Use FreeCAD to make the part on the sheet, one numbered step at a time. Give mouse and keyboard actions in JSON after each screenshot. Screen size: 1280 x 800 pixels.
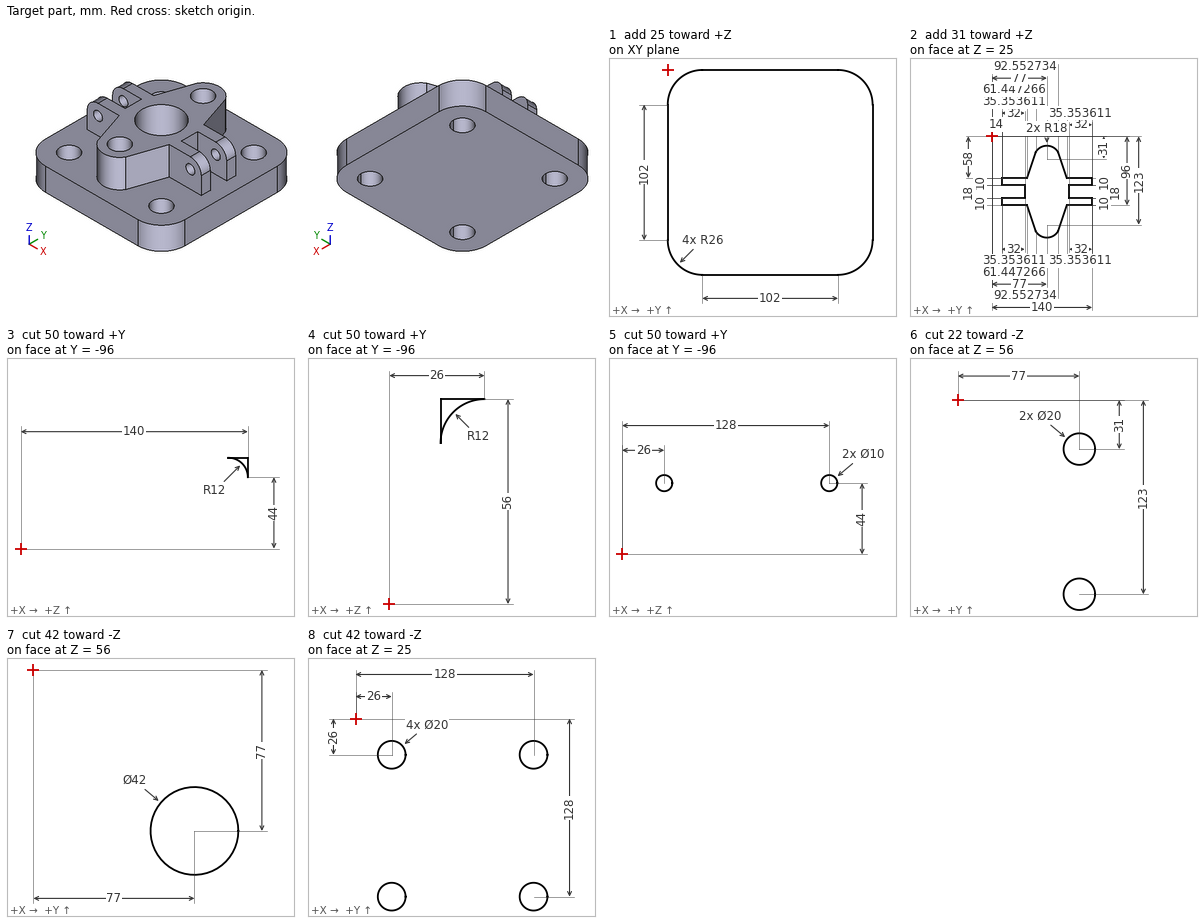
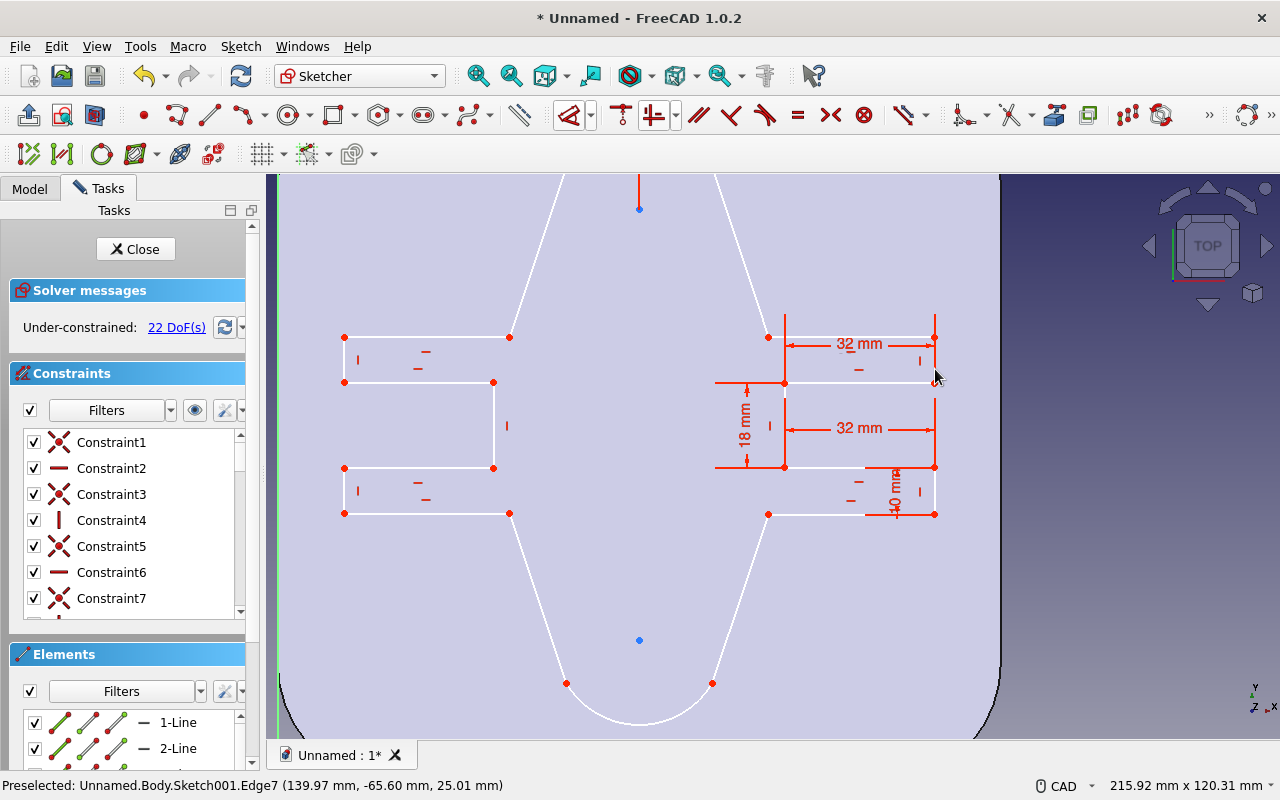
{"action": "left_click", "coordinate": [590, 116]}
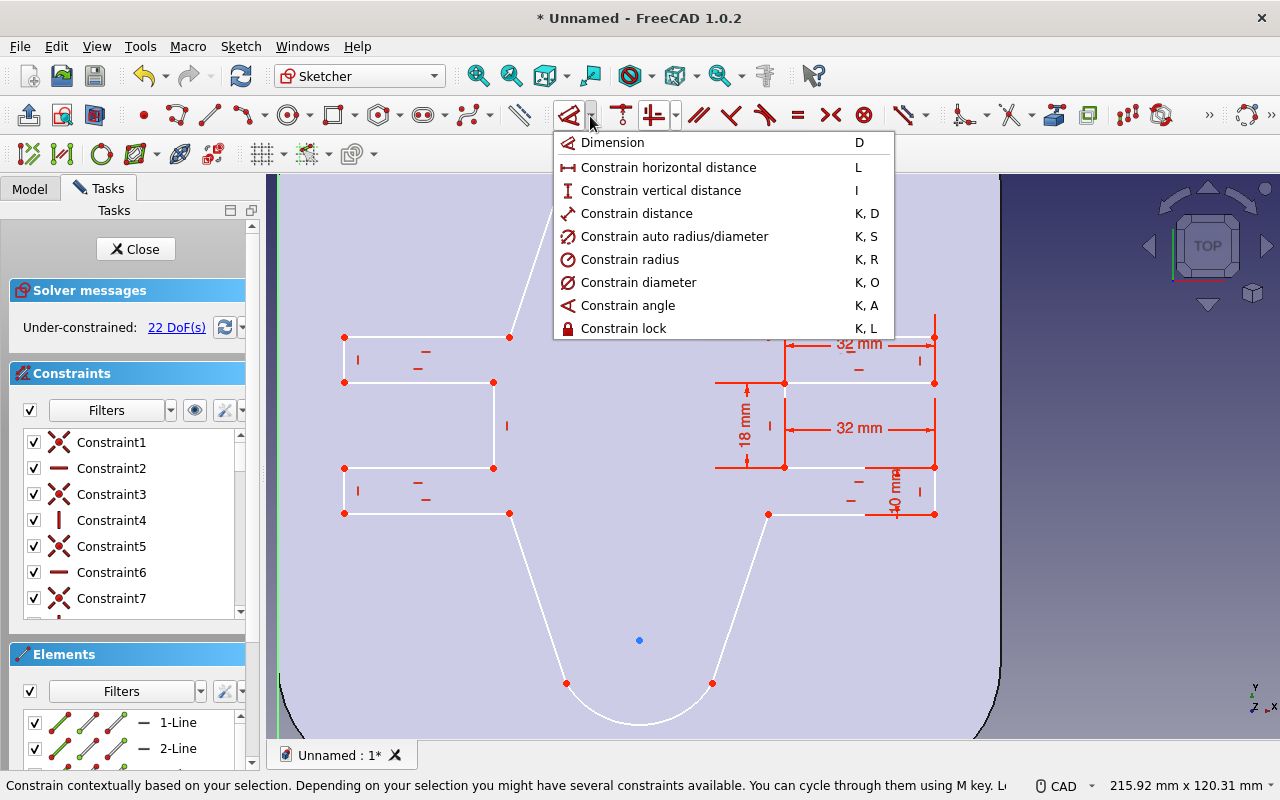
{"action": "left_click", "coordinate": [724, 190]}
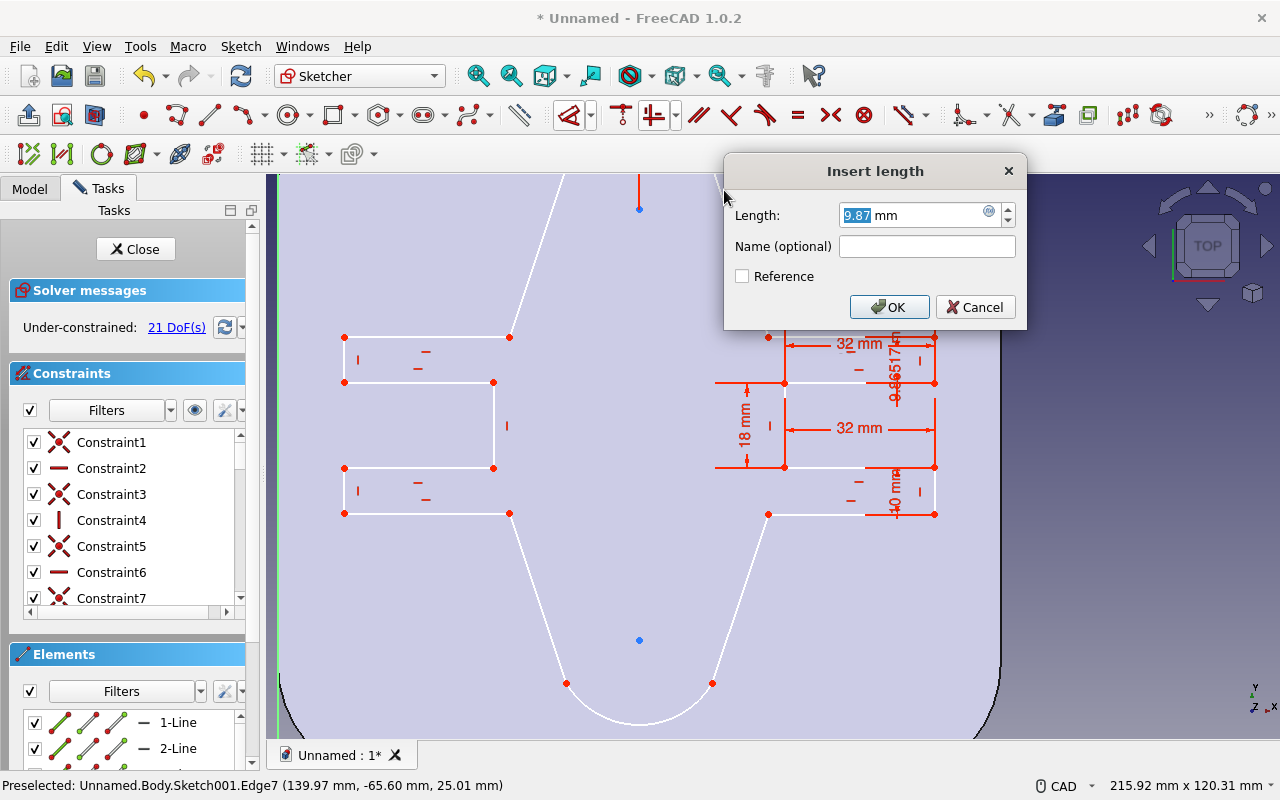
{"action": "type", "text": "10"}
{"action": "key", "text": "Return"}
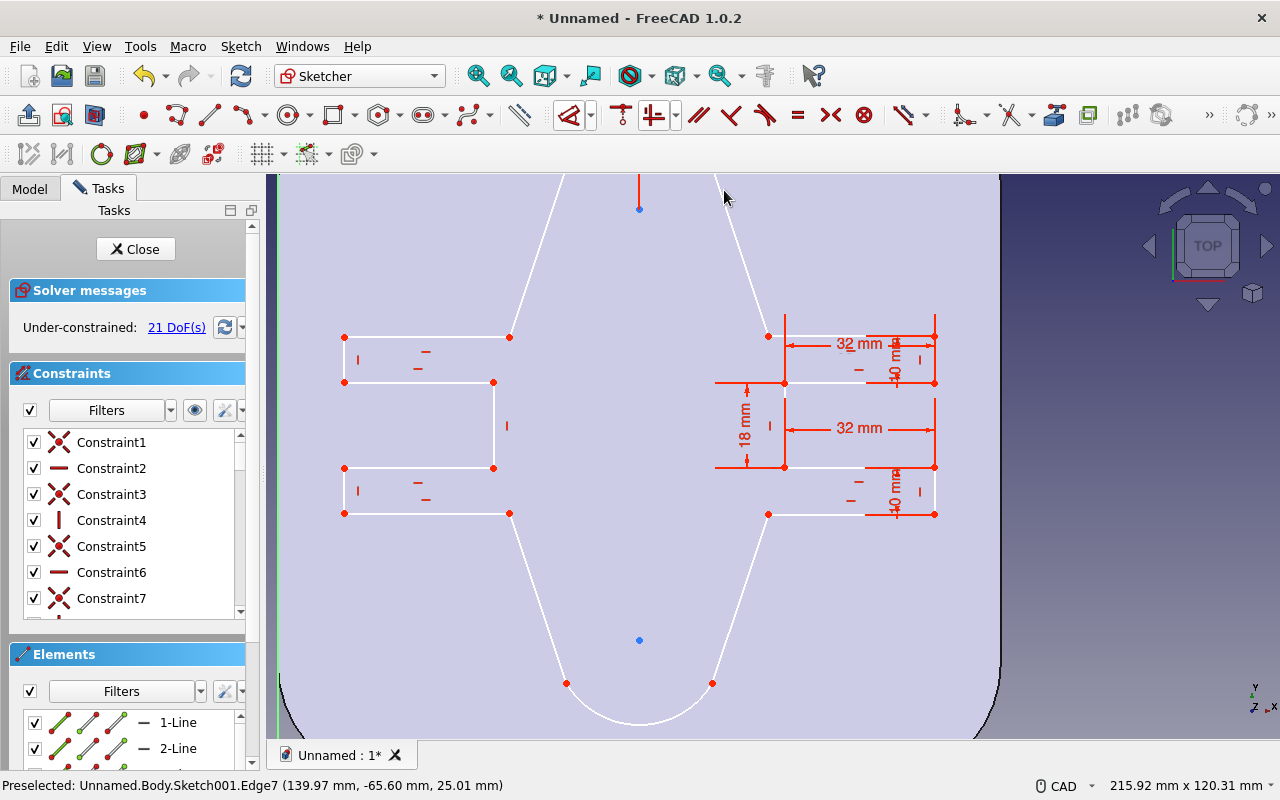
{"action": "left_click", "coordinate": [344, 351]}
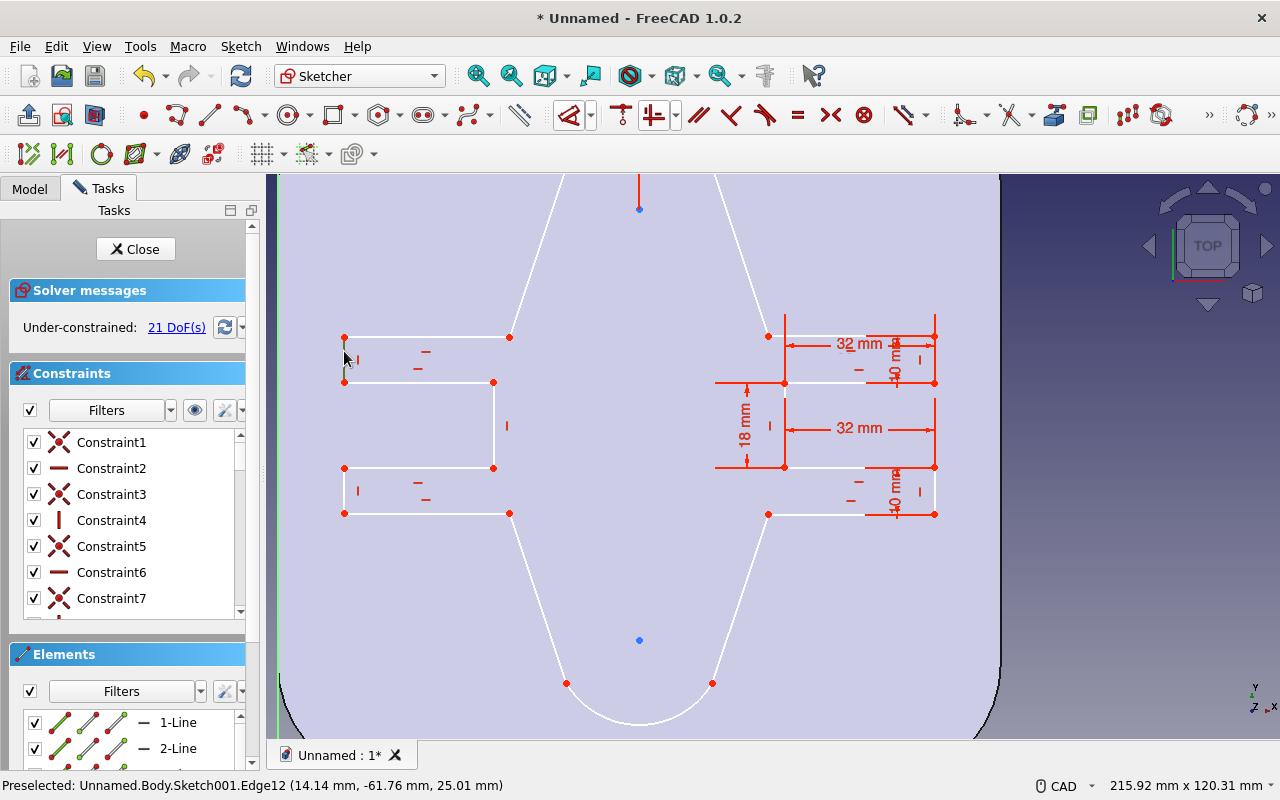
{"action": "key", "text": "i"}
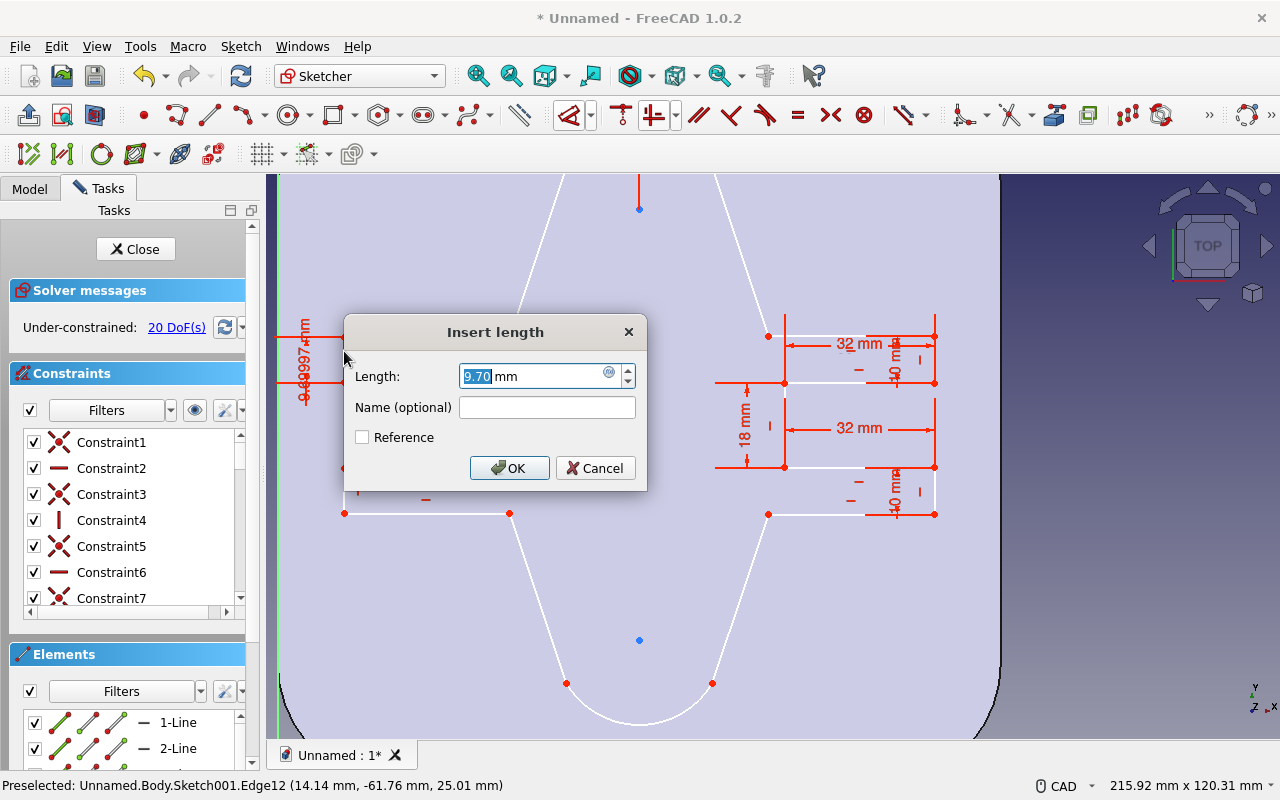
{"action": "type", "text": "10"}
{"action": "key", "text": "Return"}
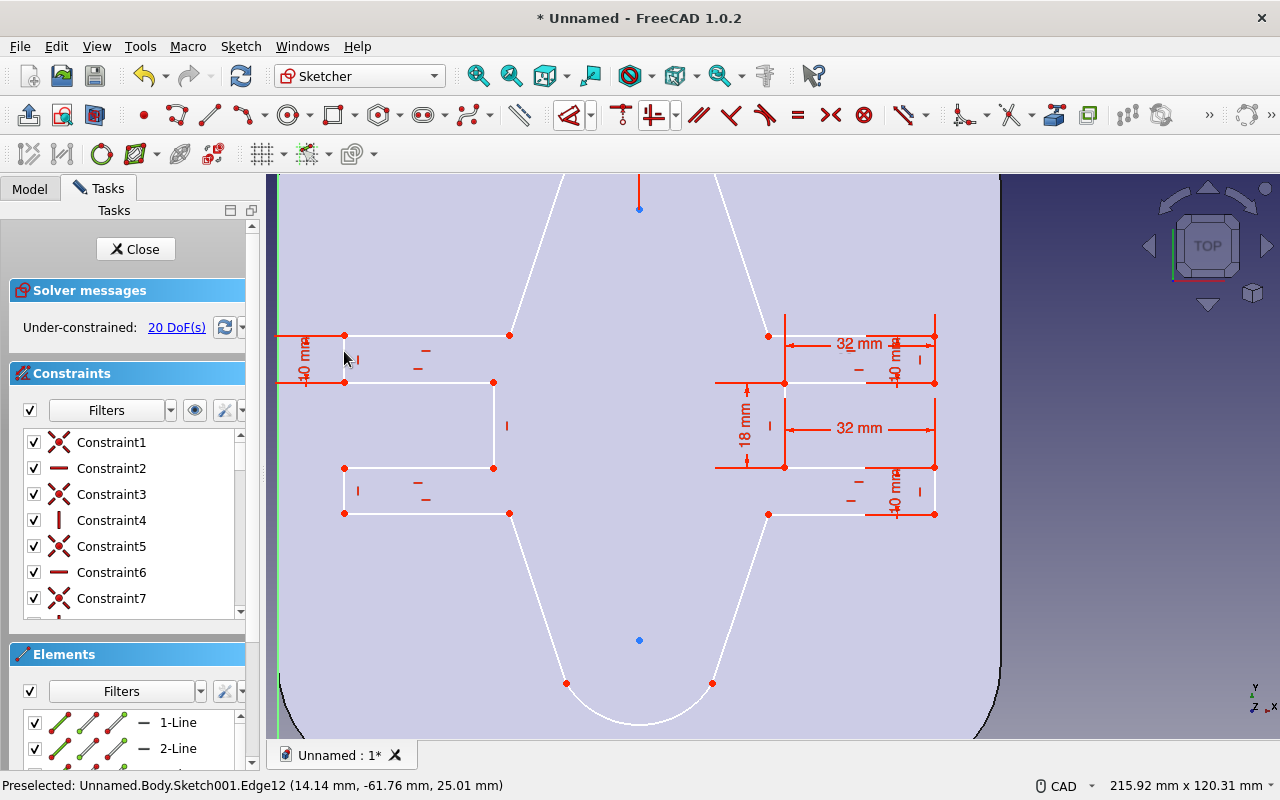
{"action": "left_click", "coordinate": [389, 383]}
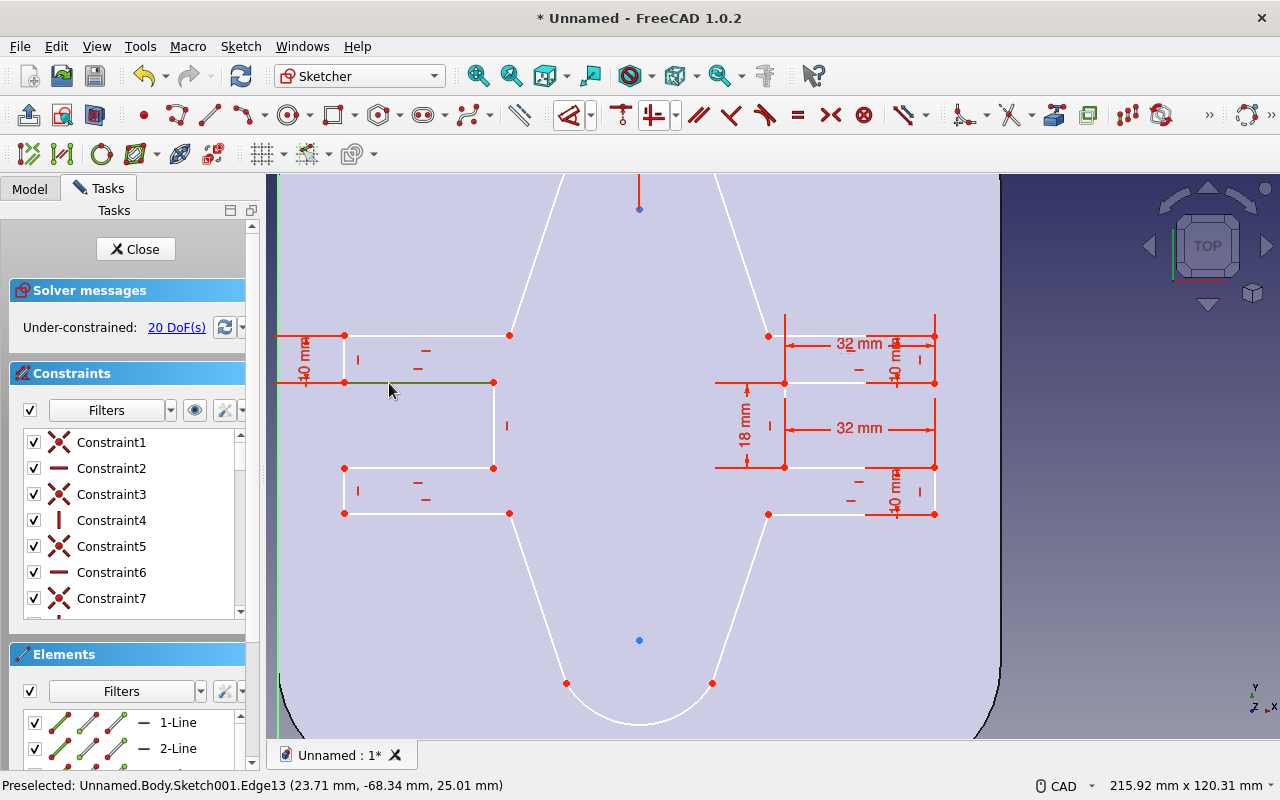
{"action": "left_click", "coordinate": [590, 116]}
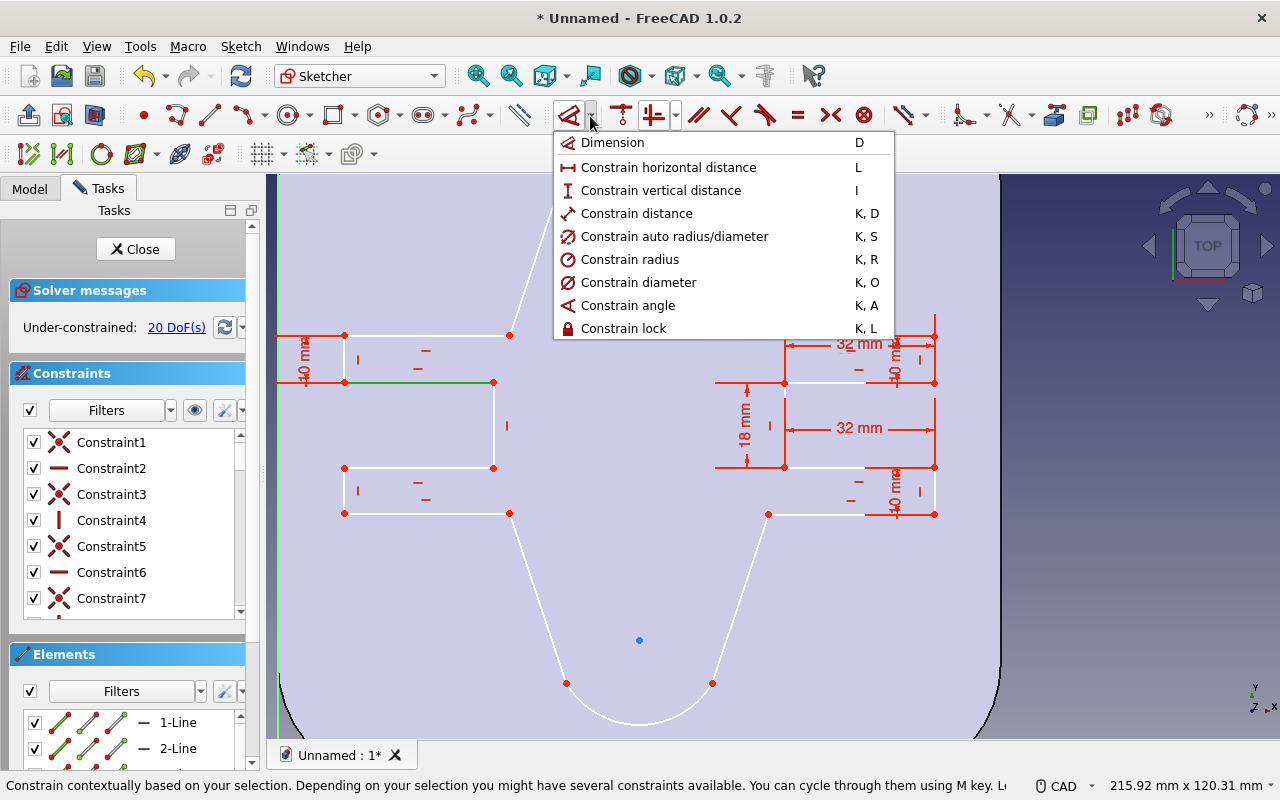
{"action": "left_click", "coordinate": [724, 168]}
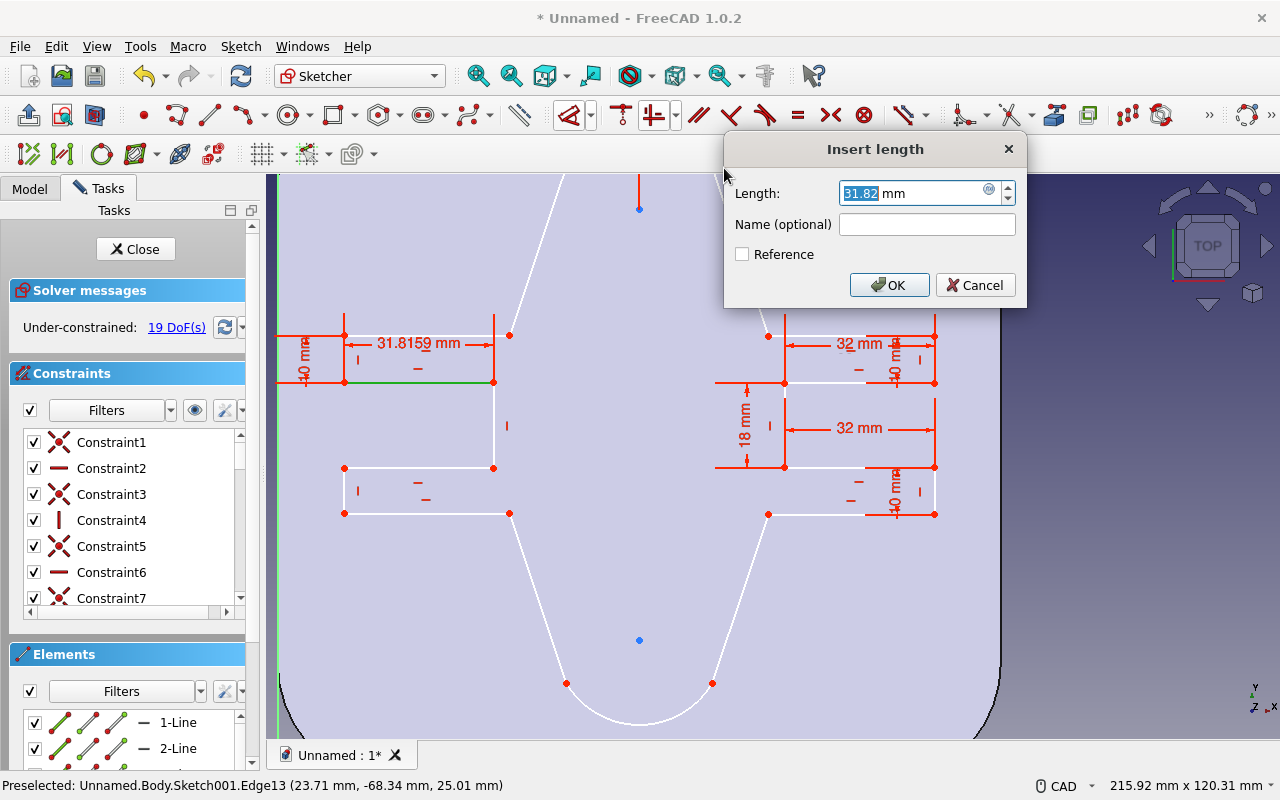
{"action": "type", "text": "32"}
{"action": "key", "text": "Return"}